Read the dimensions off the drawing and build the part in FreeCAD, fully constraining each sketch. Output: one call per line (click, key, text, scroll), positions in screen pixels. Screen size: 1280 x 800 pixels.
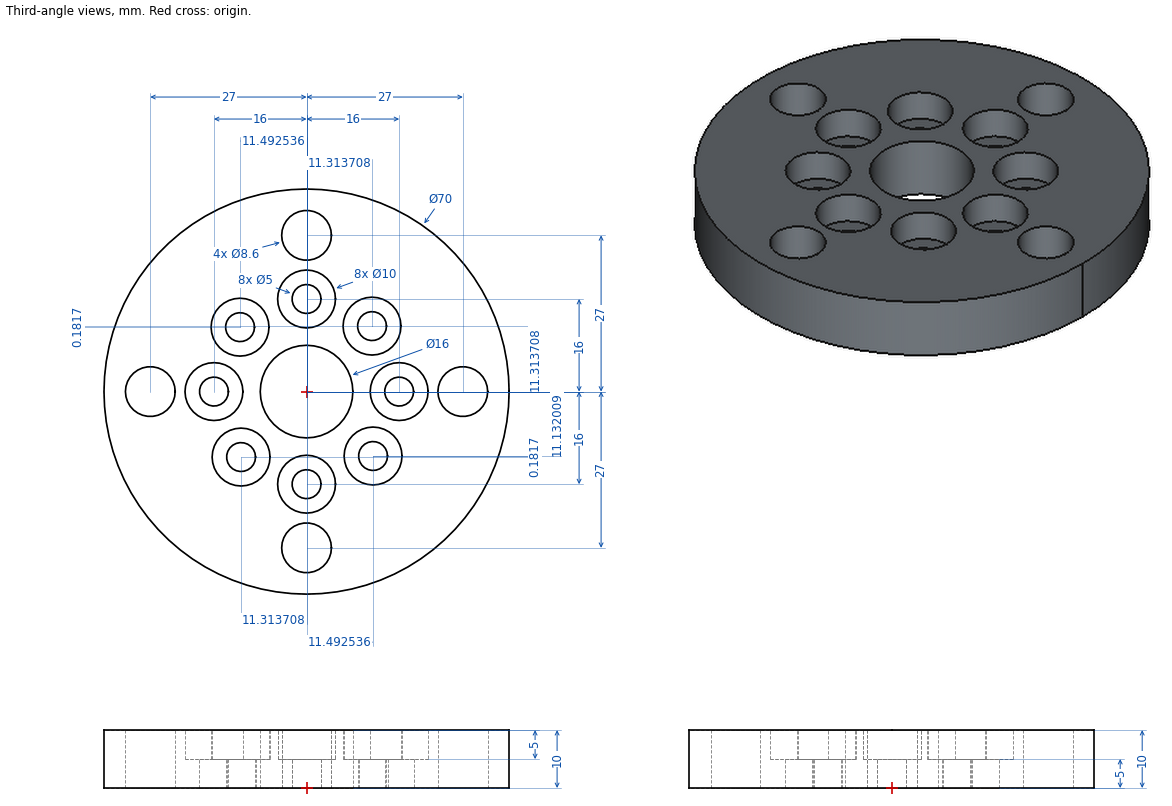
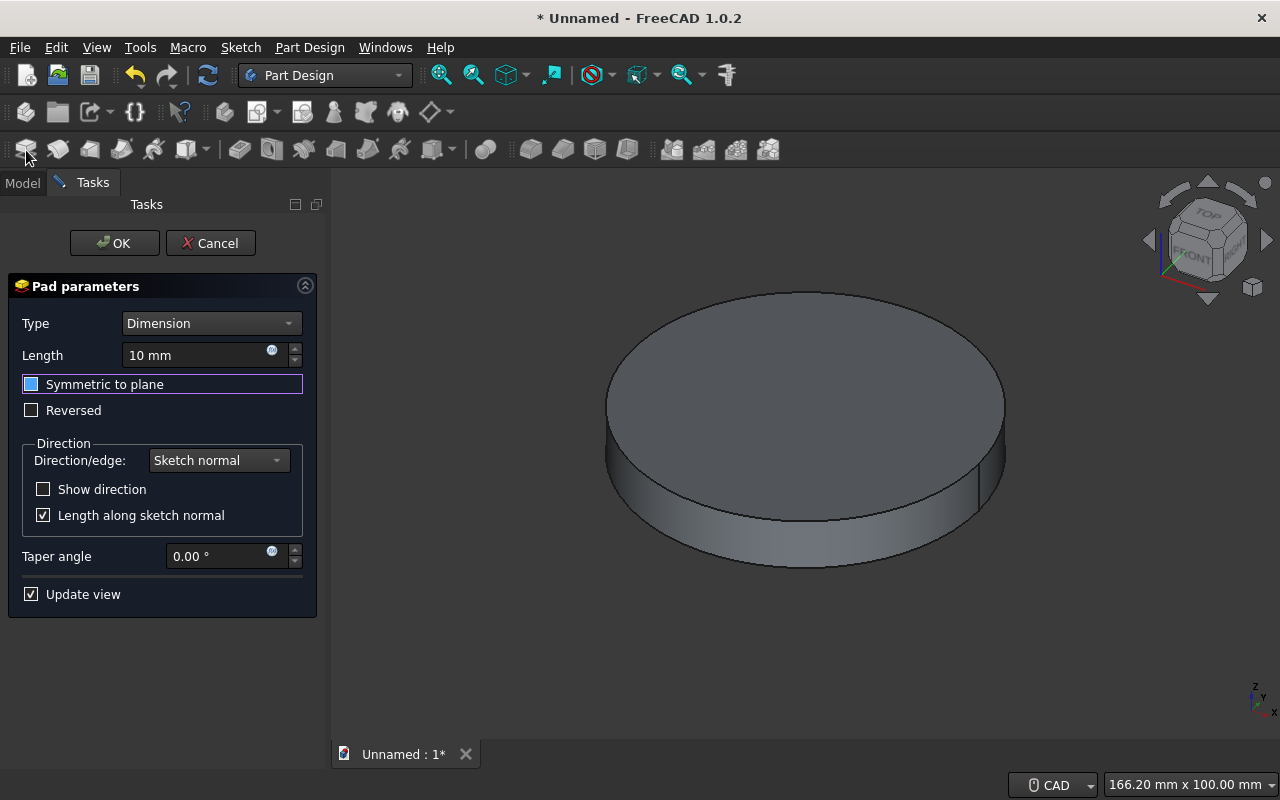
click(115, 243)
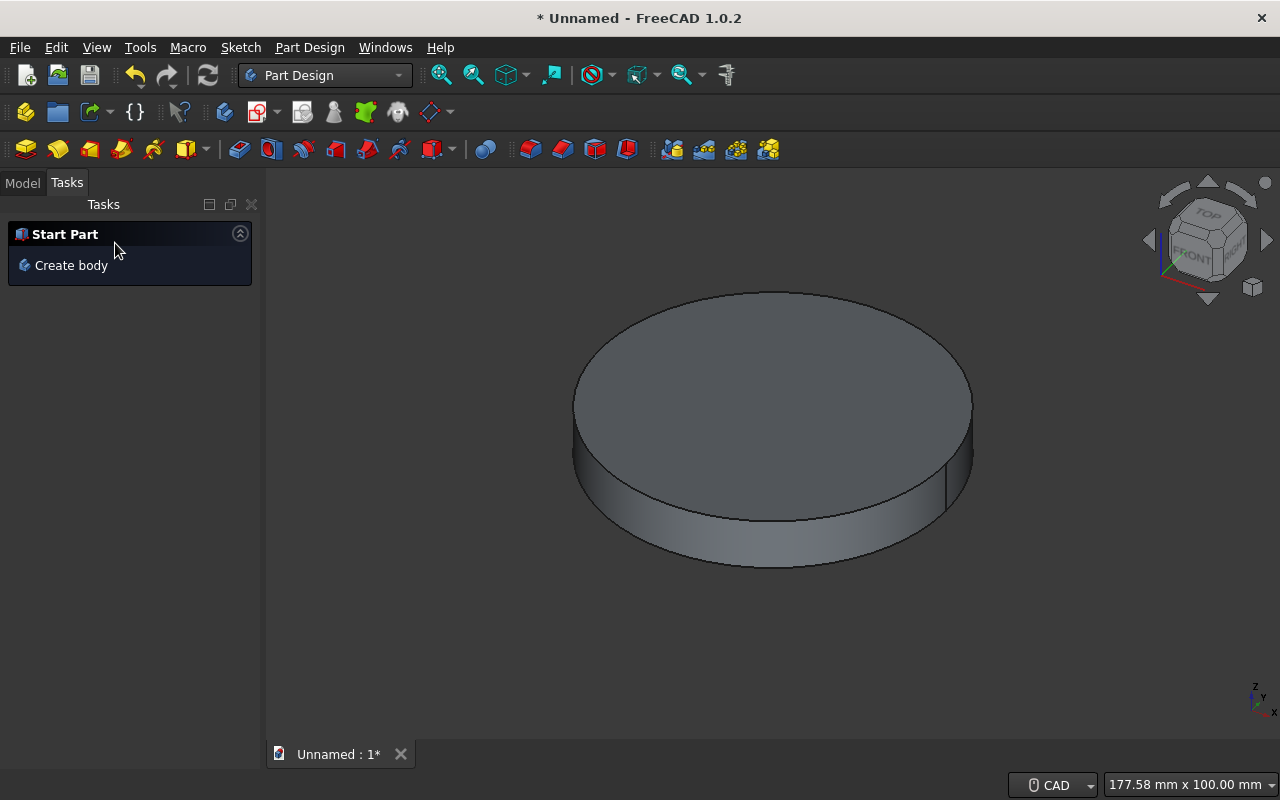
click(773, 406)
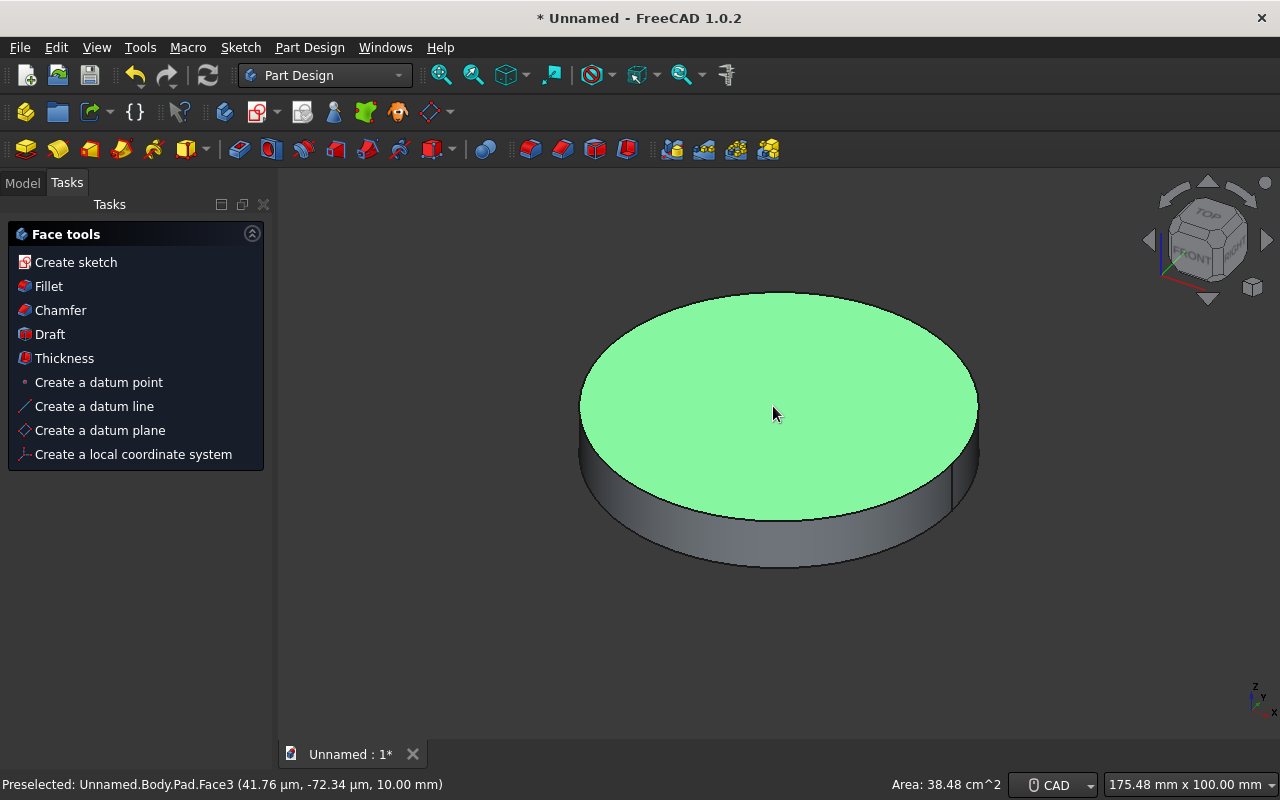
click(258, 112)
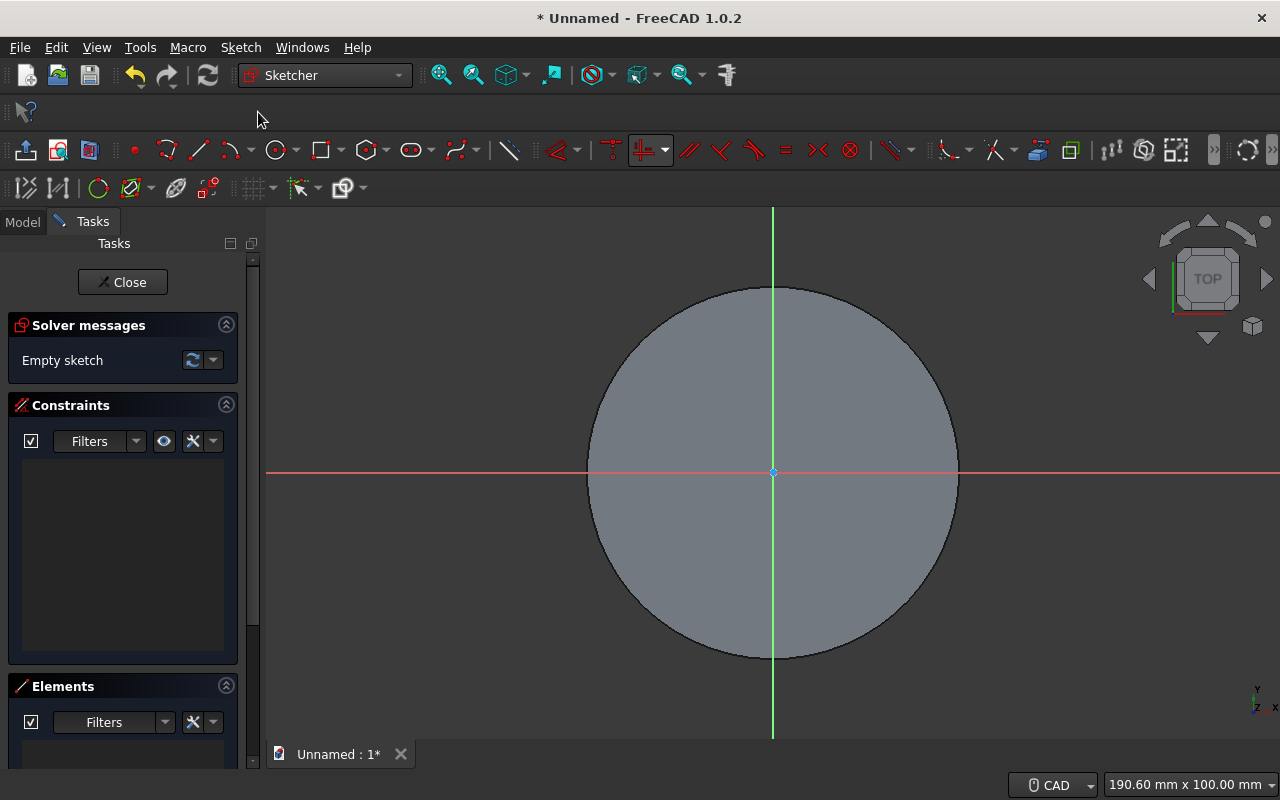
scroll(795, 473, up, 7)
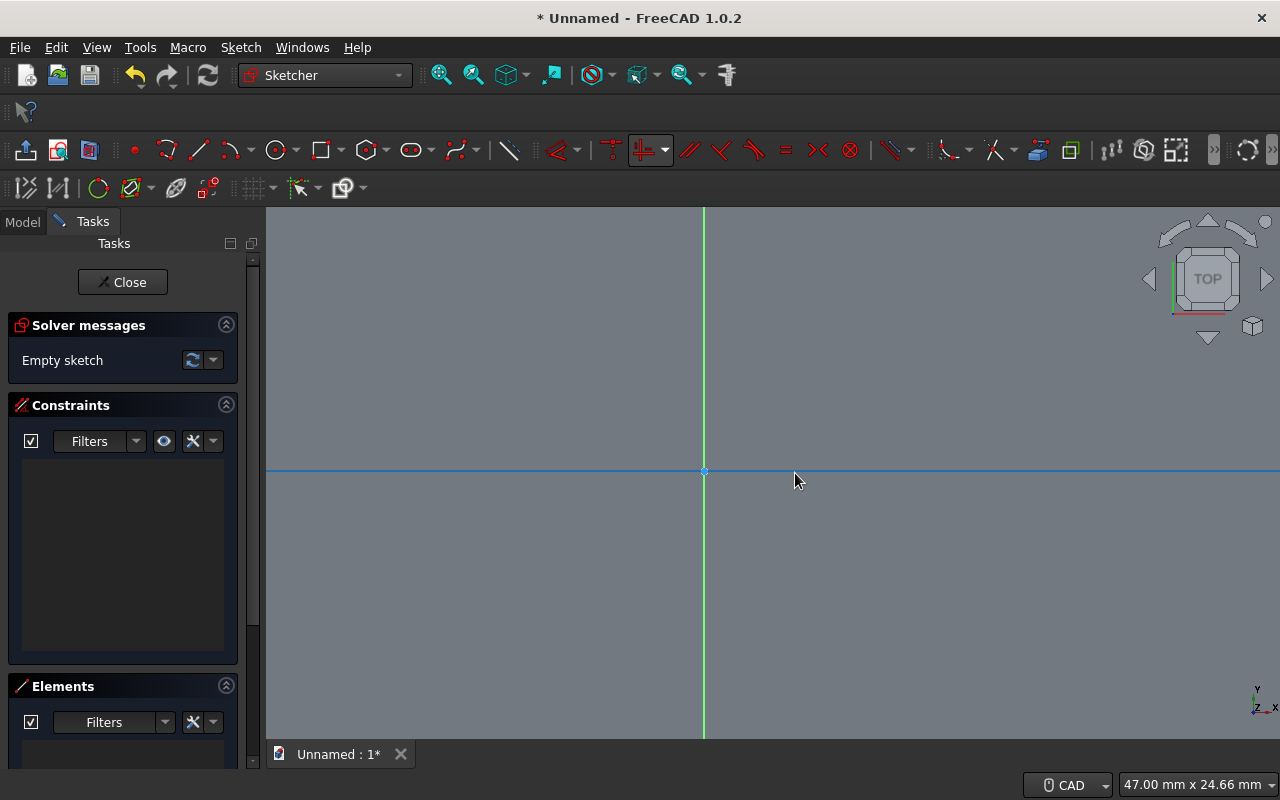
click(276, 150)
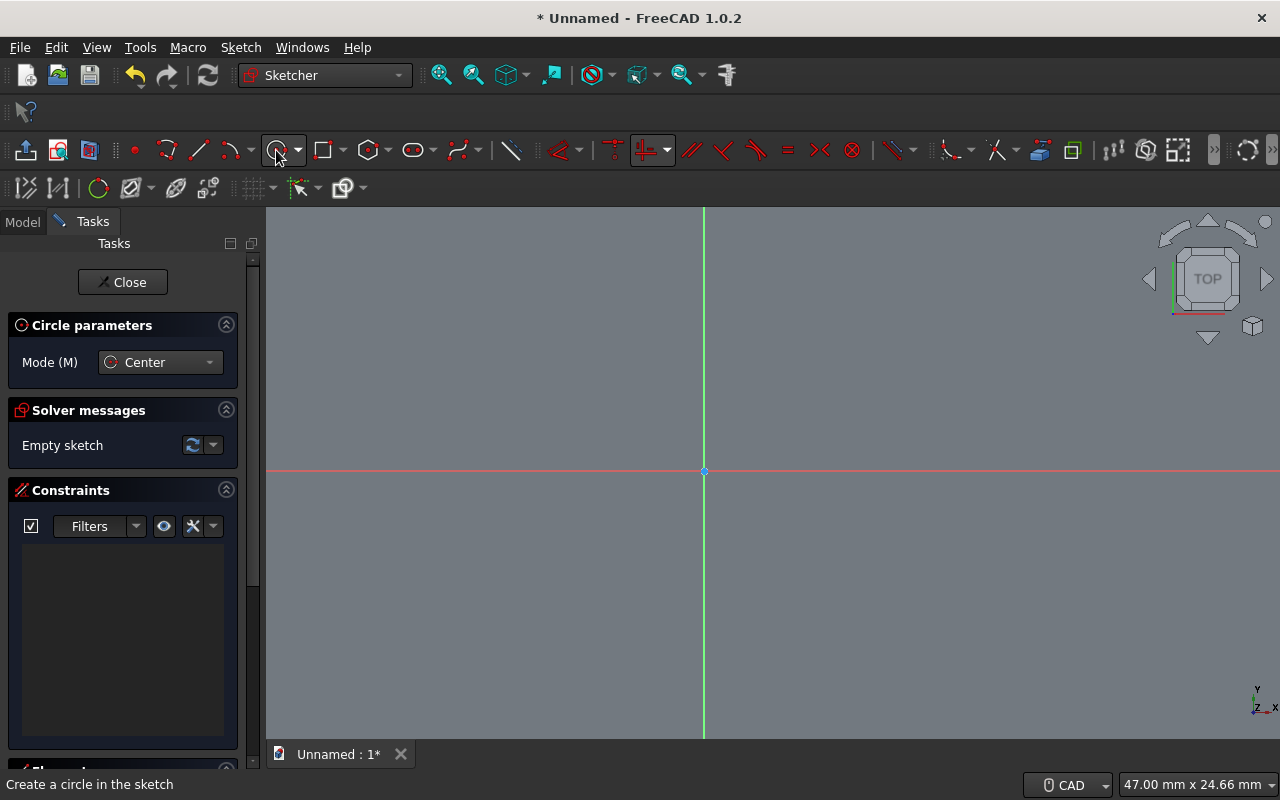
click(704, 471)
move(826, 349)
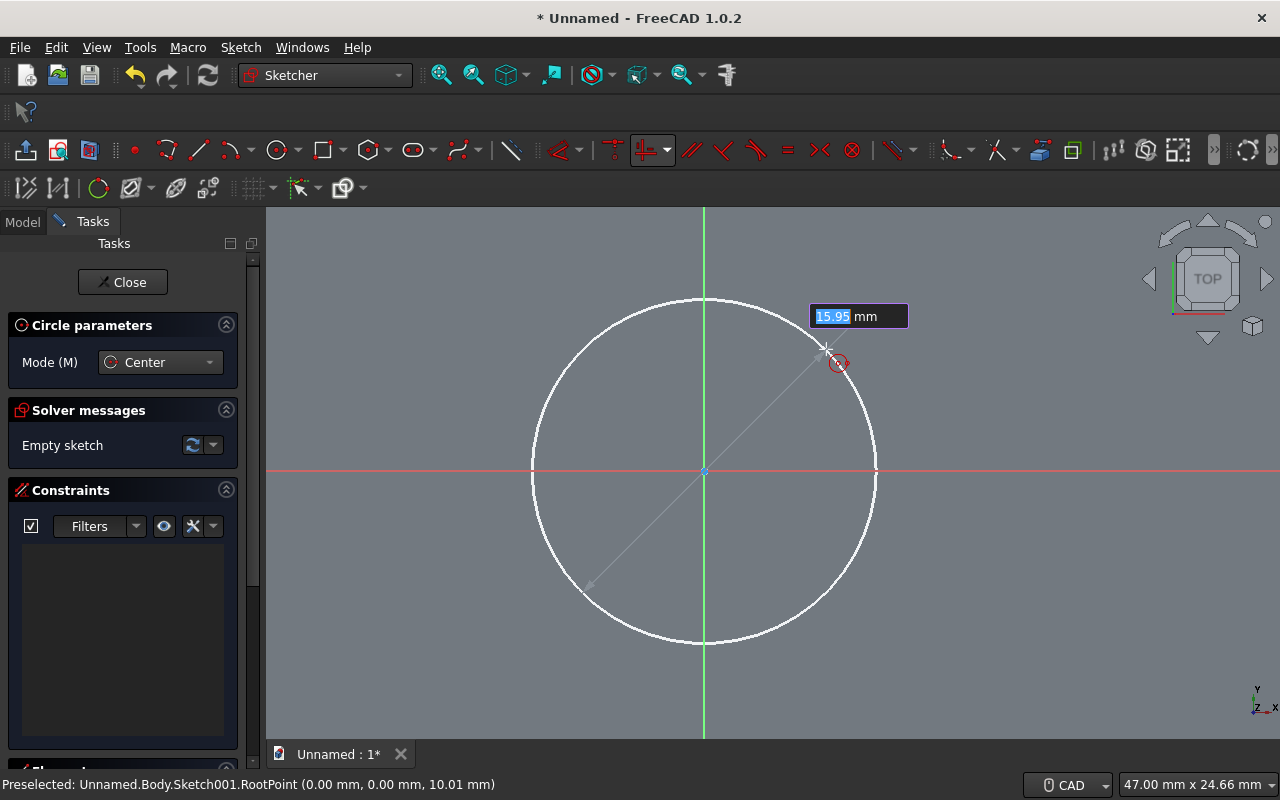
text(16)
key(Return)
key(Escape)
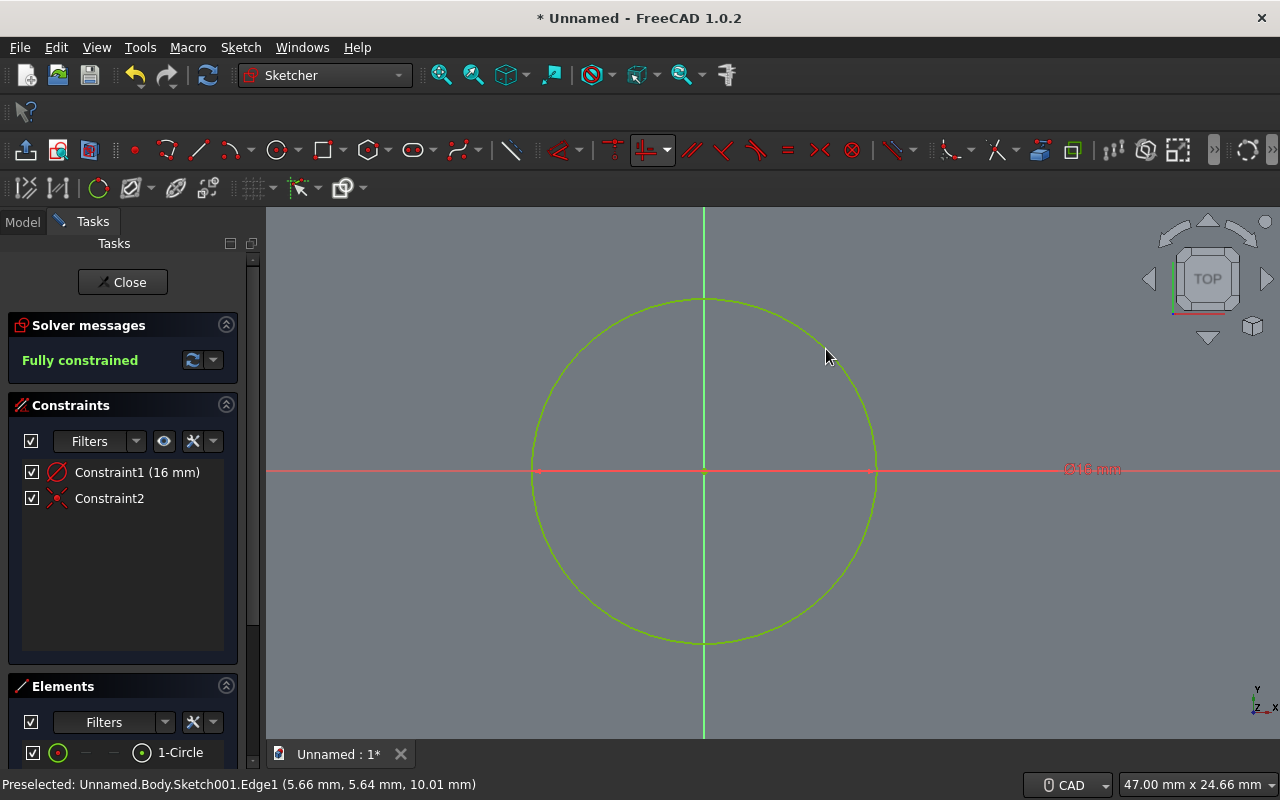
click(123, 282)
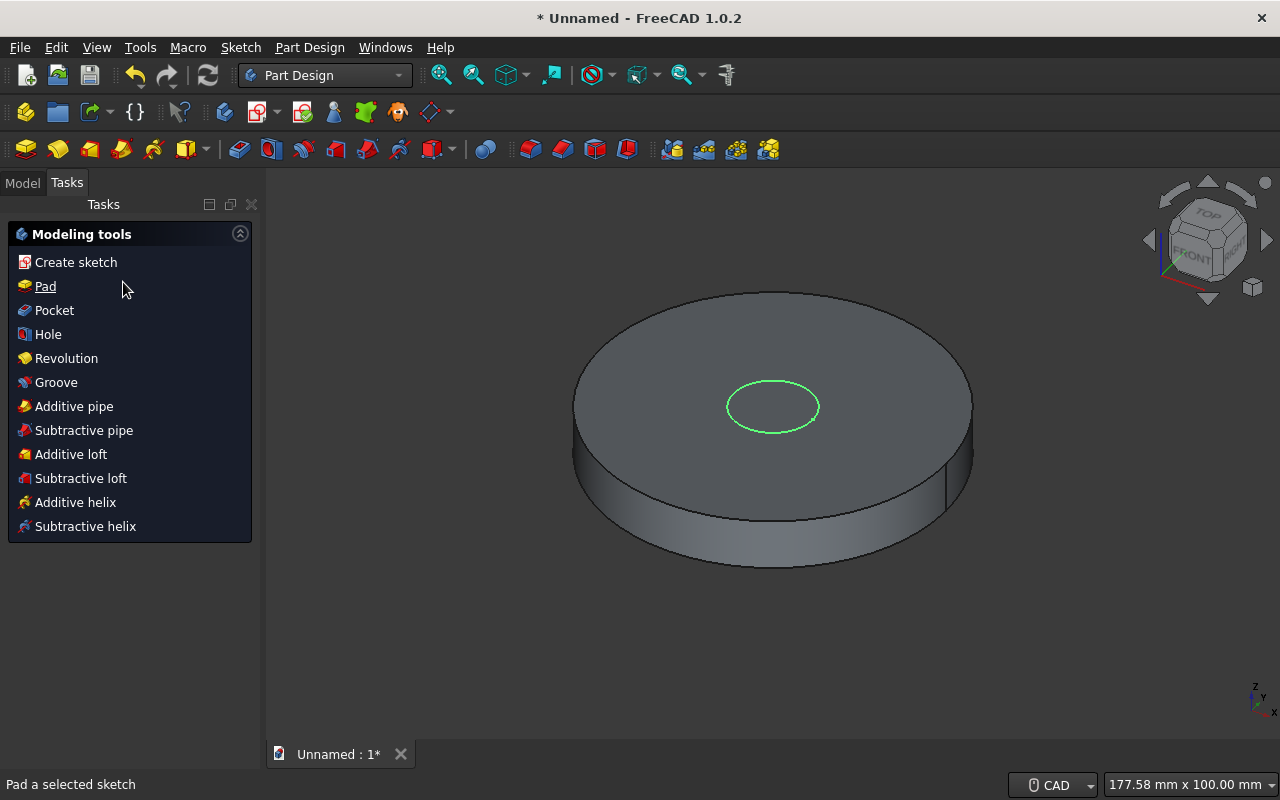
click(240, 150)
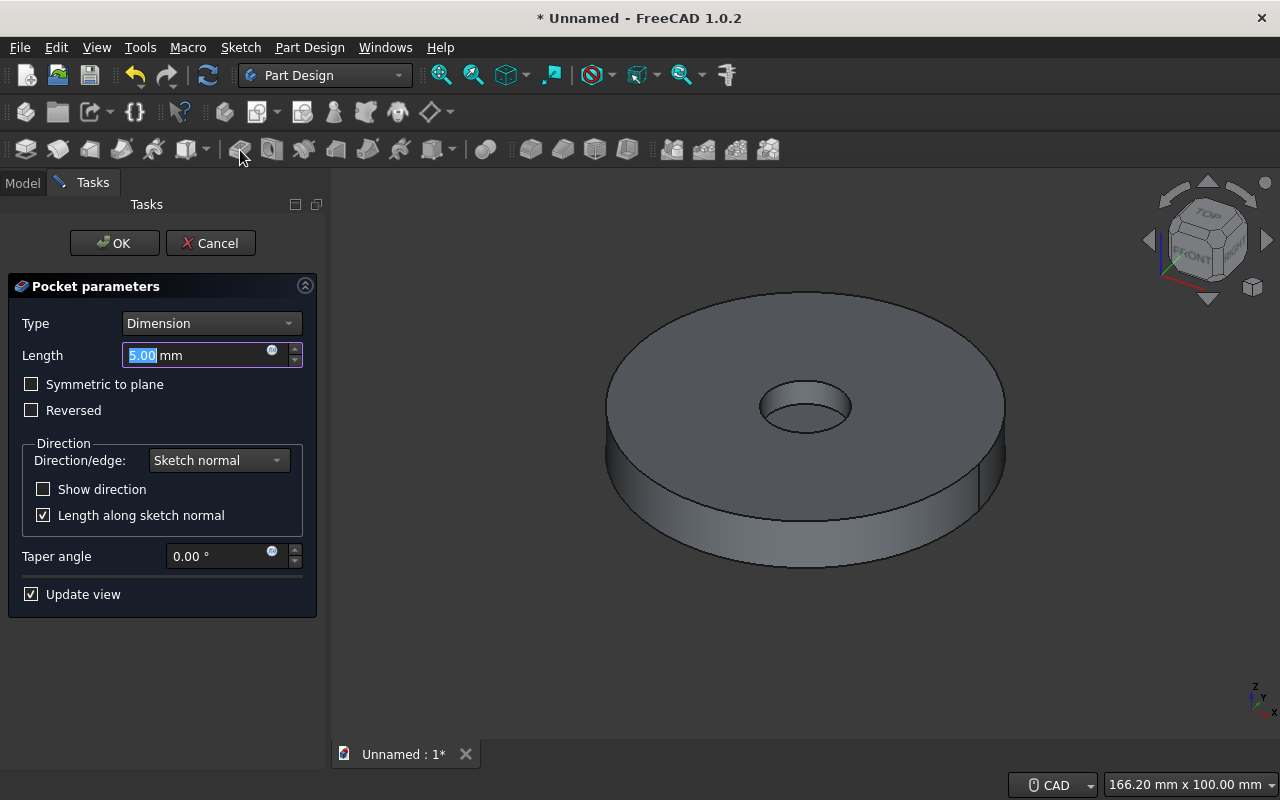
text(10)
key(Tab)